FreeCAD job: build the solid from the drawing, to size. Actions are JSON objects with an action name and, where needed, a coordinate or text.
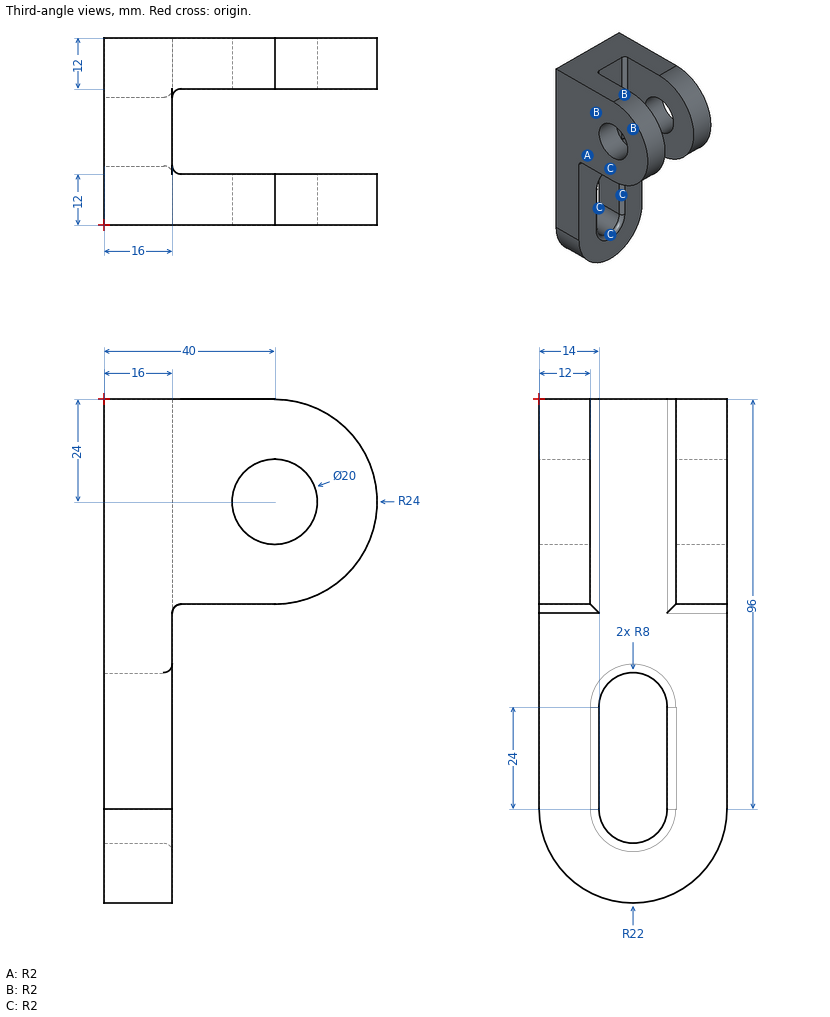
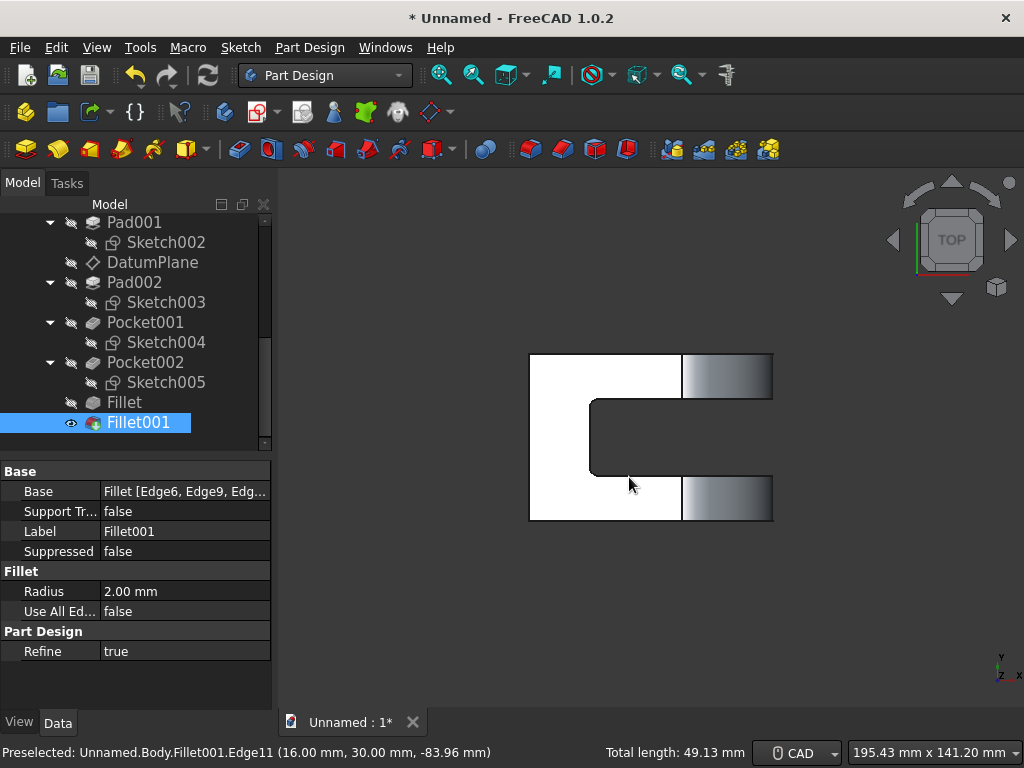
{"action": "left_click", "coordinate": [442, 76]}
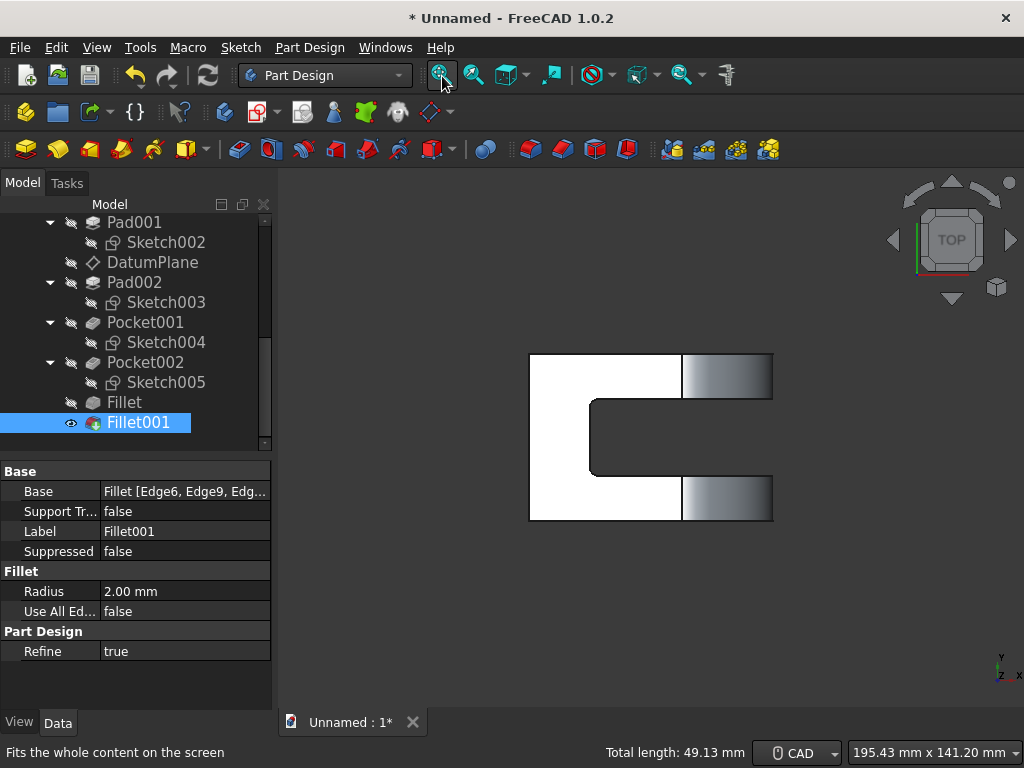
{"action": "key", "text": "0"}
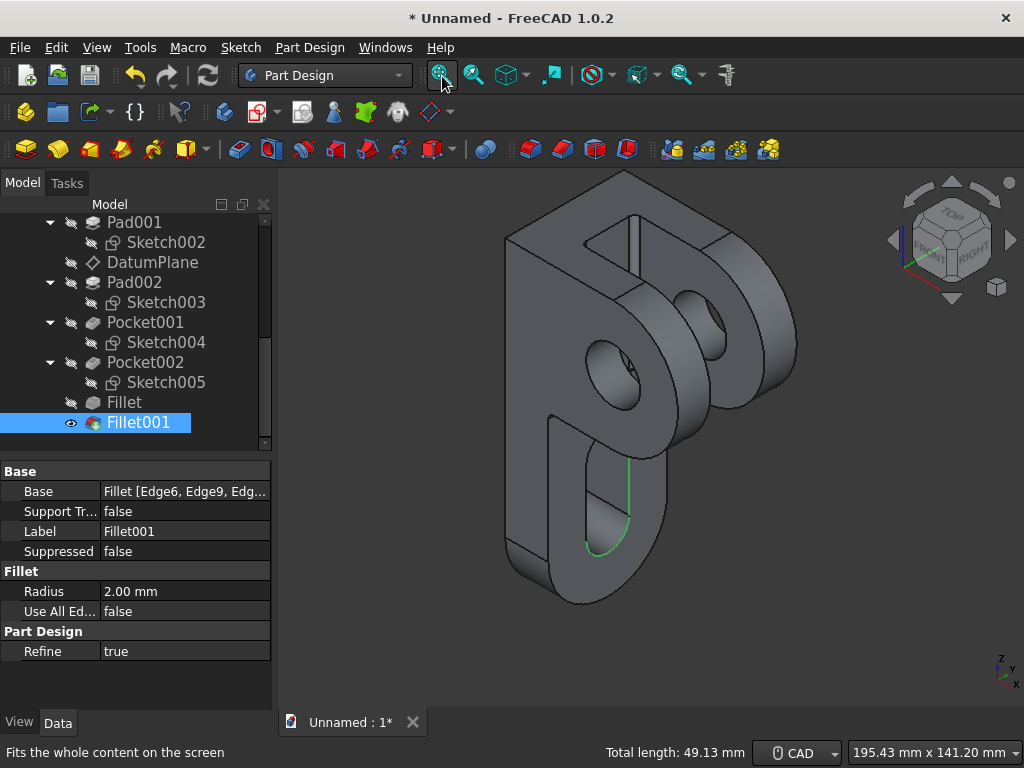
{"action": "key", "text": "1"}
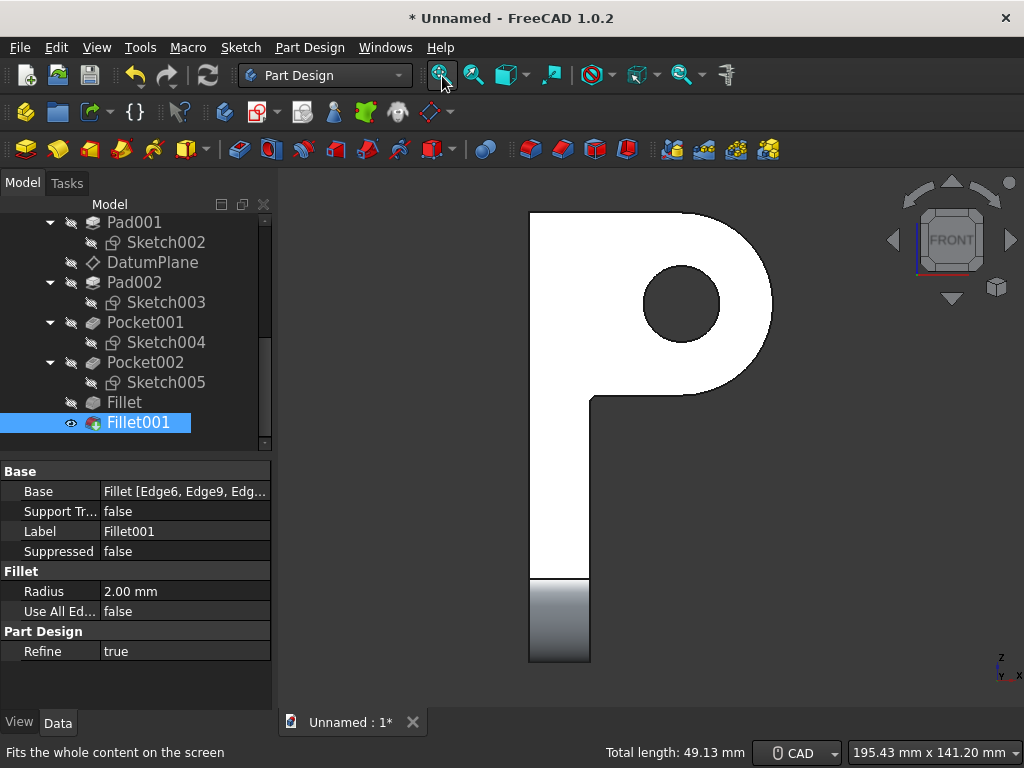
{"action": "key", "text": "3"}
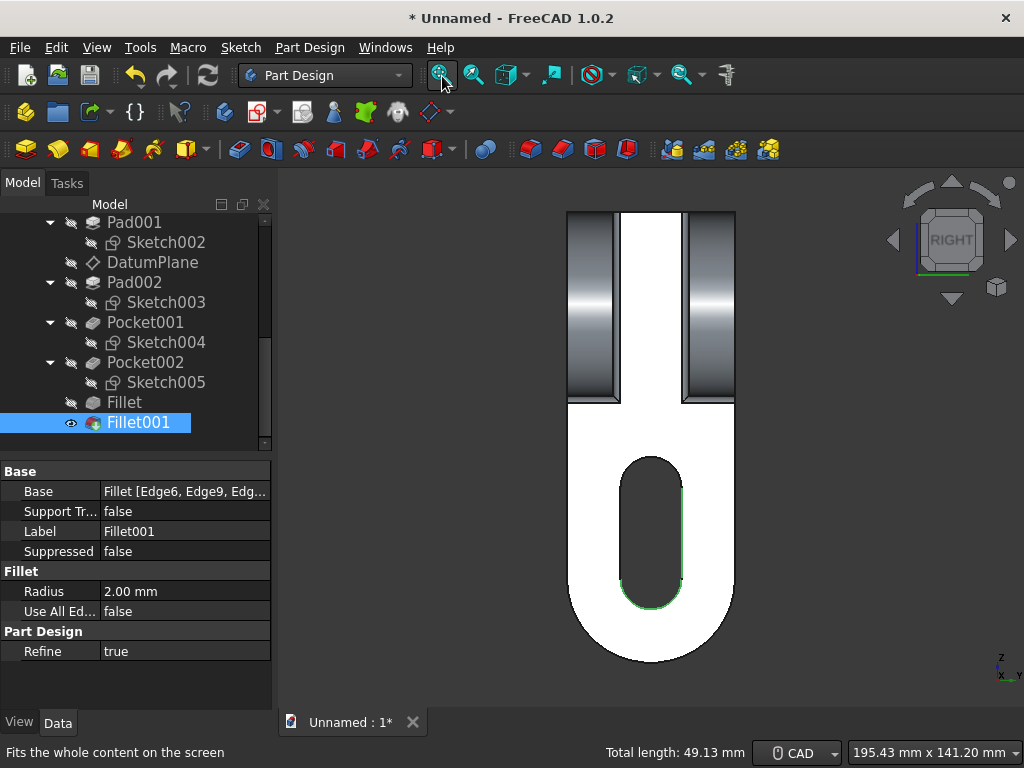
{"action": "left_click", "coordinate": [651, 456], "text": "ctrl"}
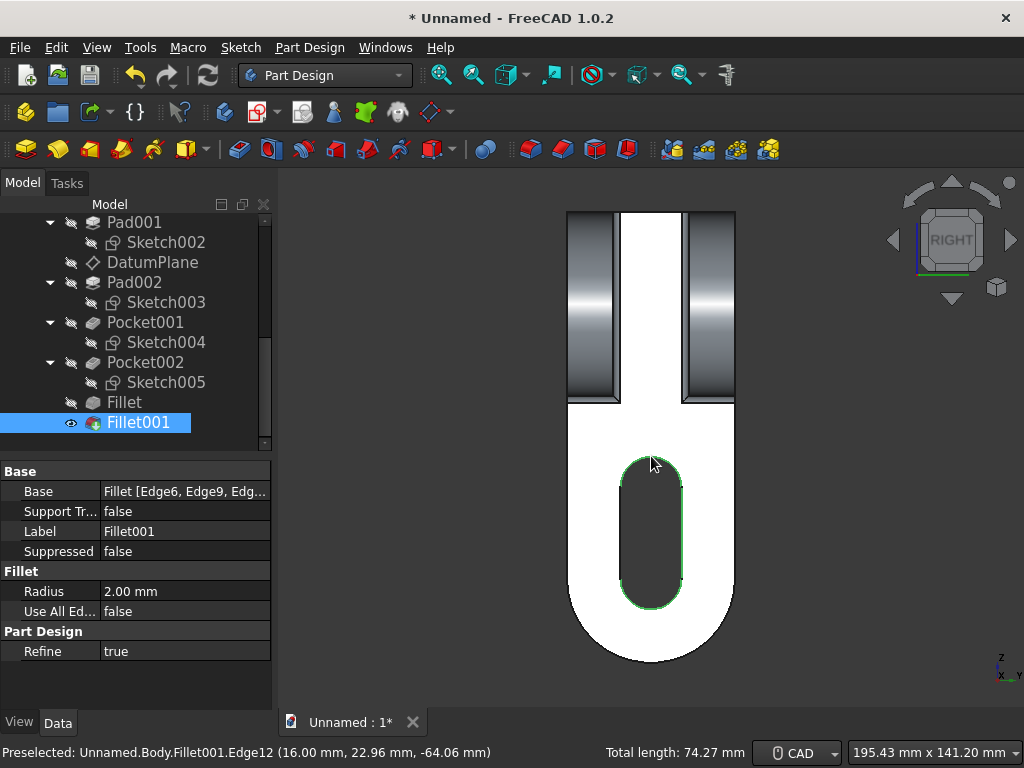
{"action": "left_click", "coordinate": [620, 532], "text": "ctrl"}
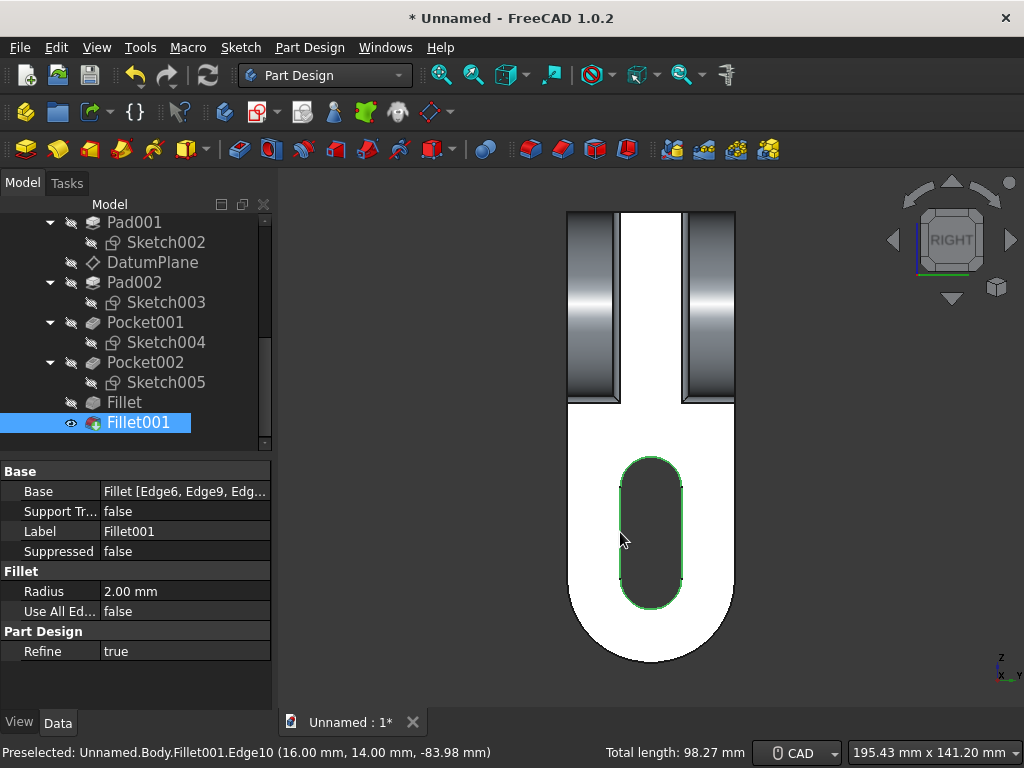
{"action": "left_click", "coordinate": [532, 150]}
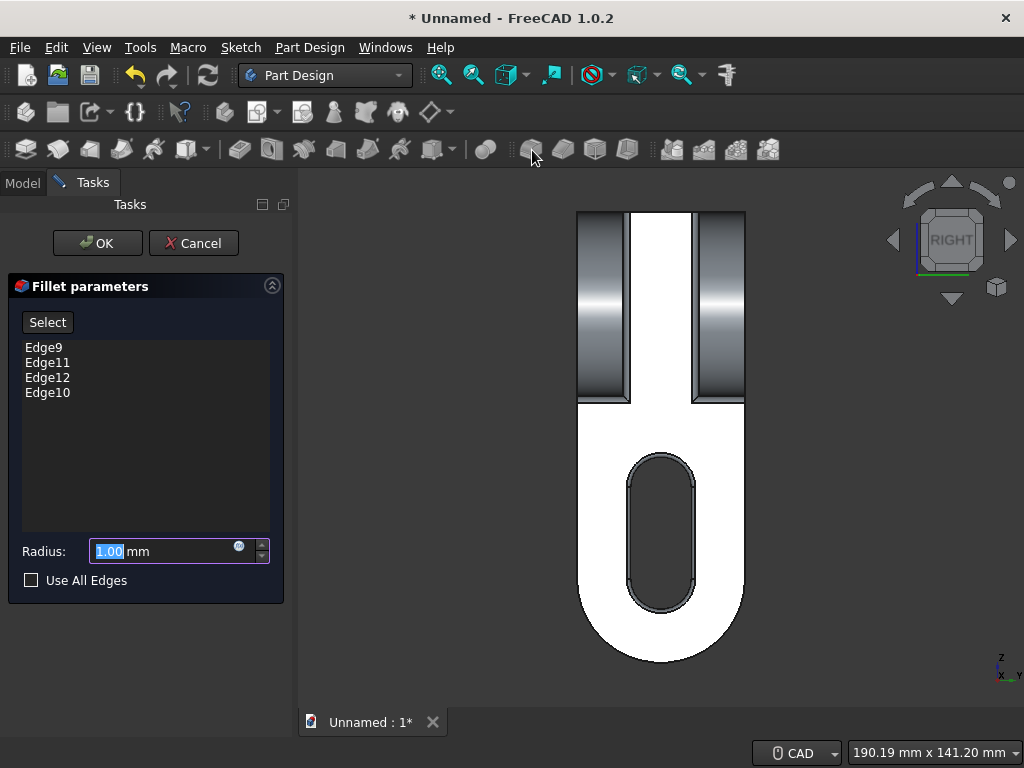
{"action": "type", "text": "2"}
{"action": "key", "text": "Tab"}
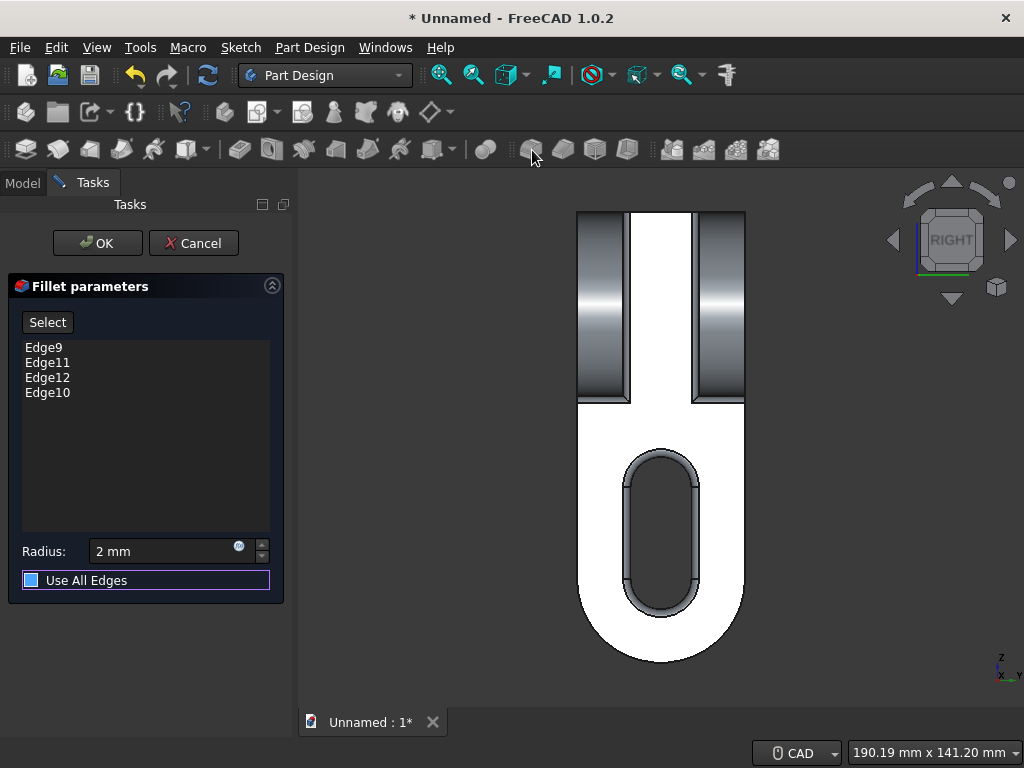
{"action": "left_click", "coordinate": [98, 243]}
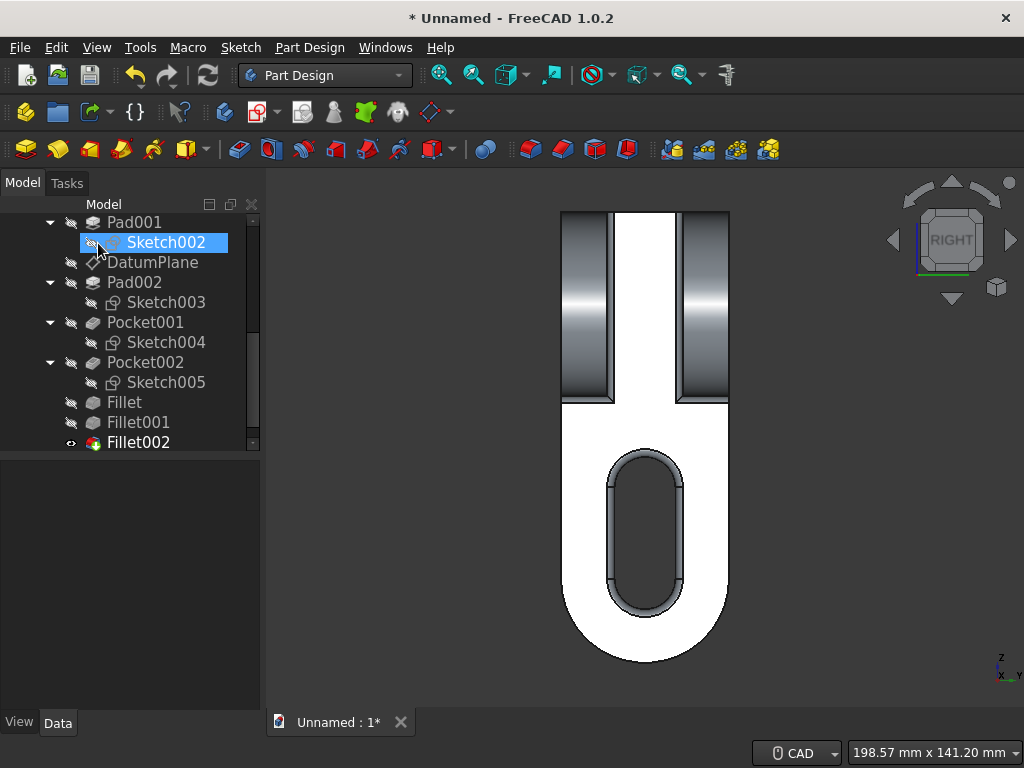
{"action": "key", "text": "0"}